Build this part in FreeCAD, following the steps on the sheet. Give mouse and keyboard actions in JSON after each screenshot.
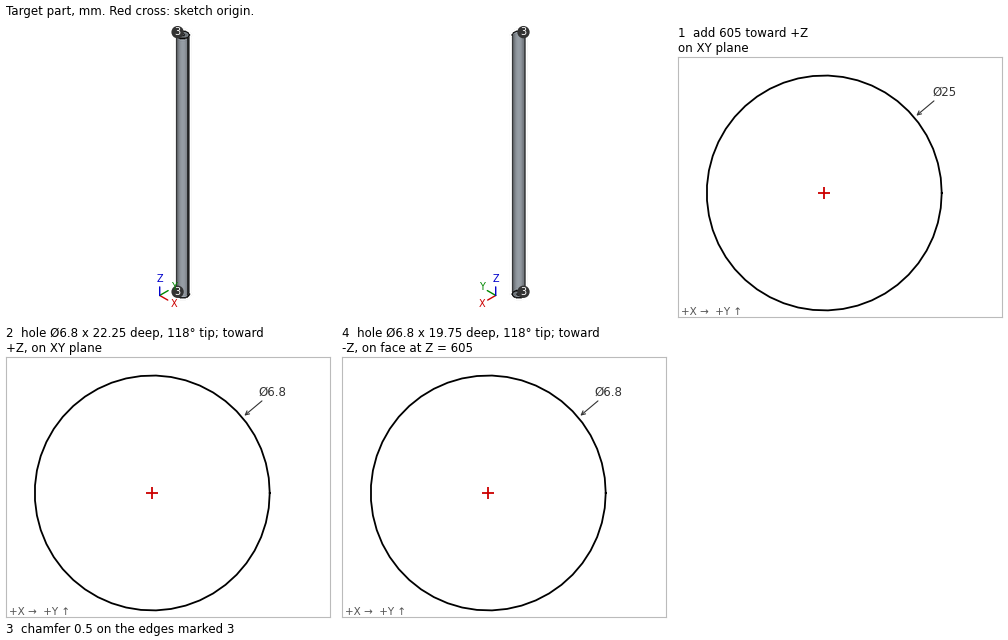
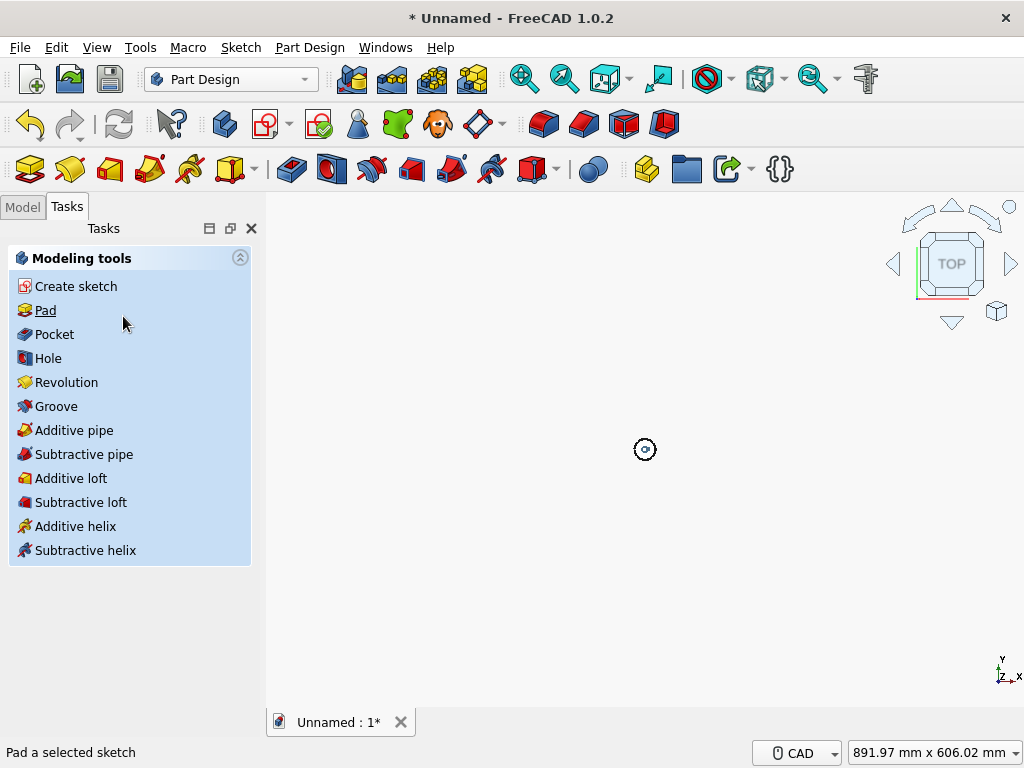
{"action": "left_click", "coordinate": [332, 170]}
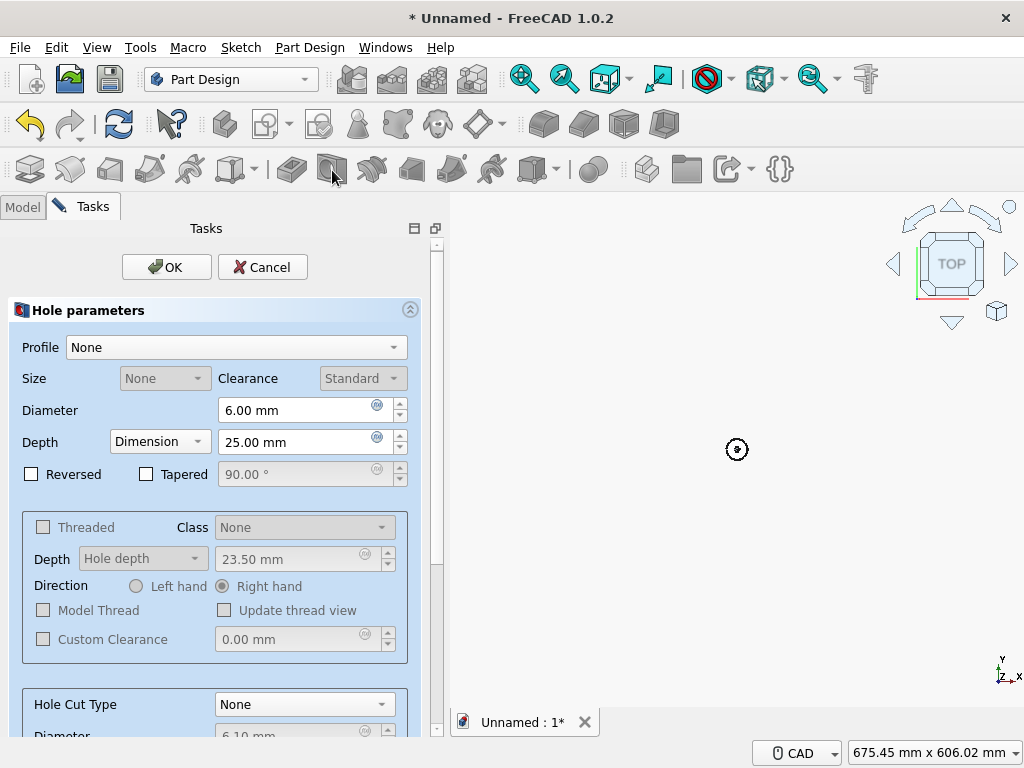
{"action": "triple_click", "coordinate": [305, 410]}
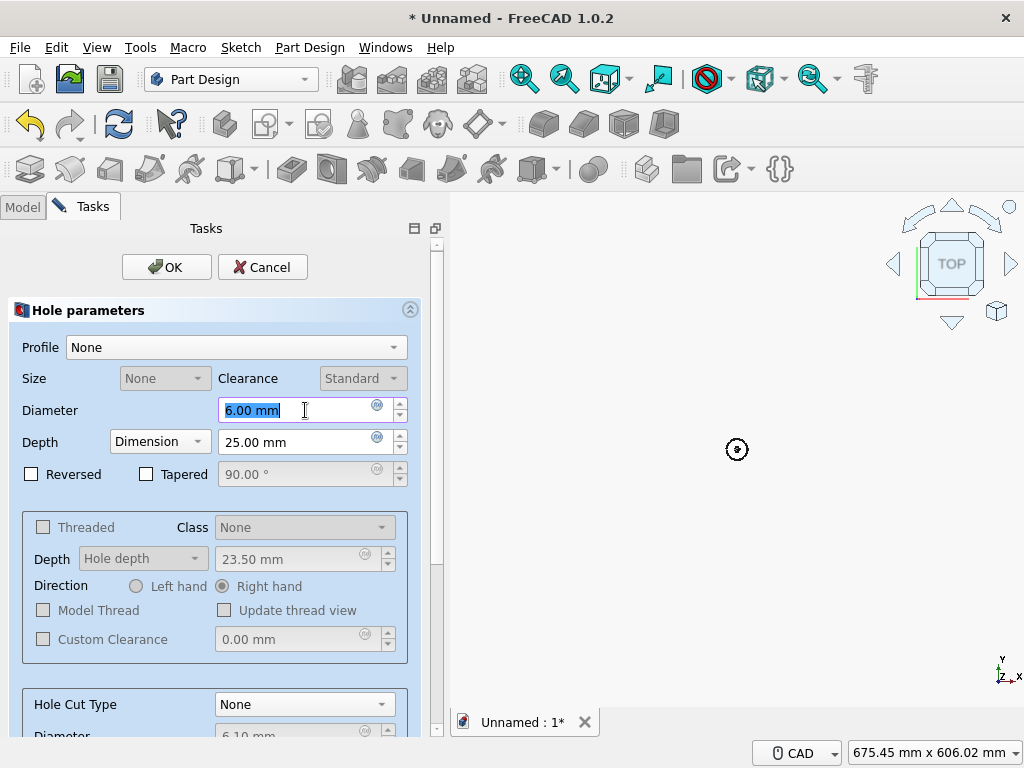
{"action": "type", "text": "6.8"}
{"action": "key", "text": "Tab"}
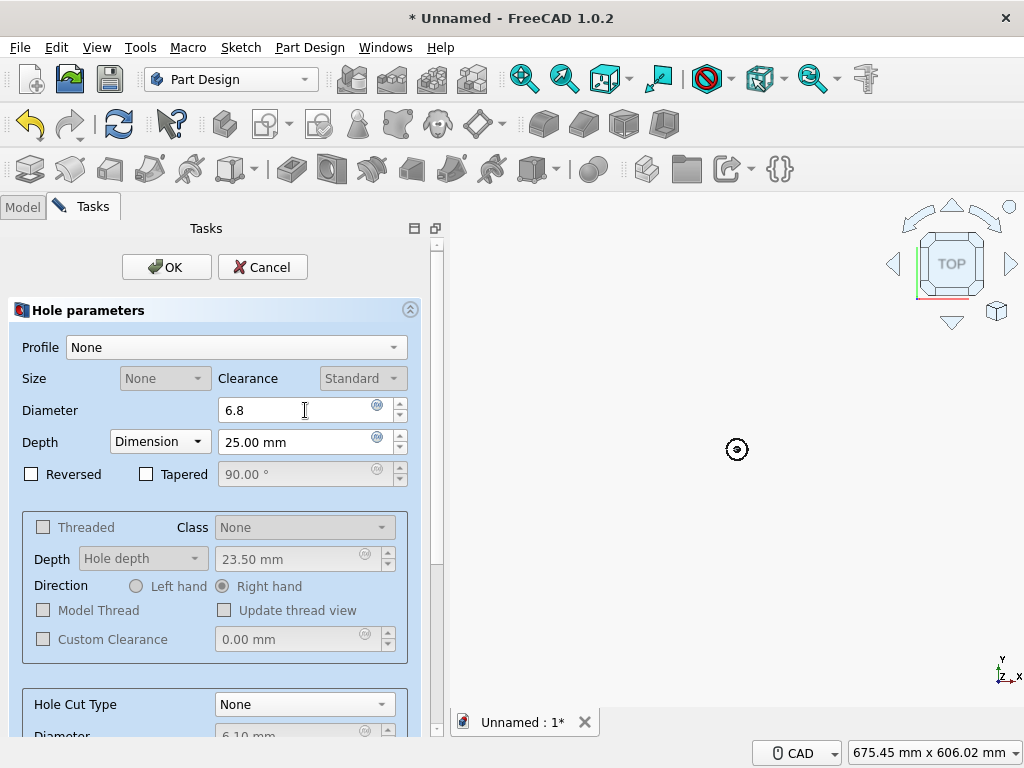
{"action": "triple_click", "coordinate": [305, 442]}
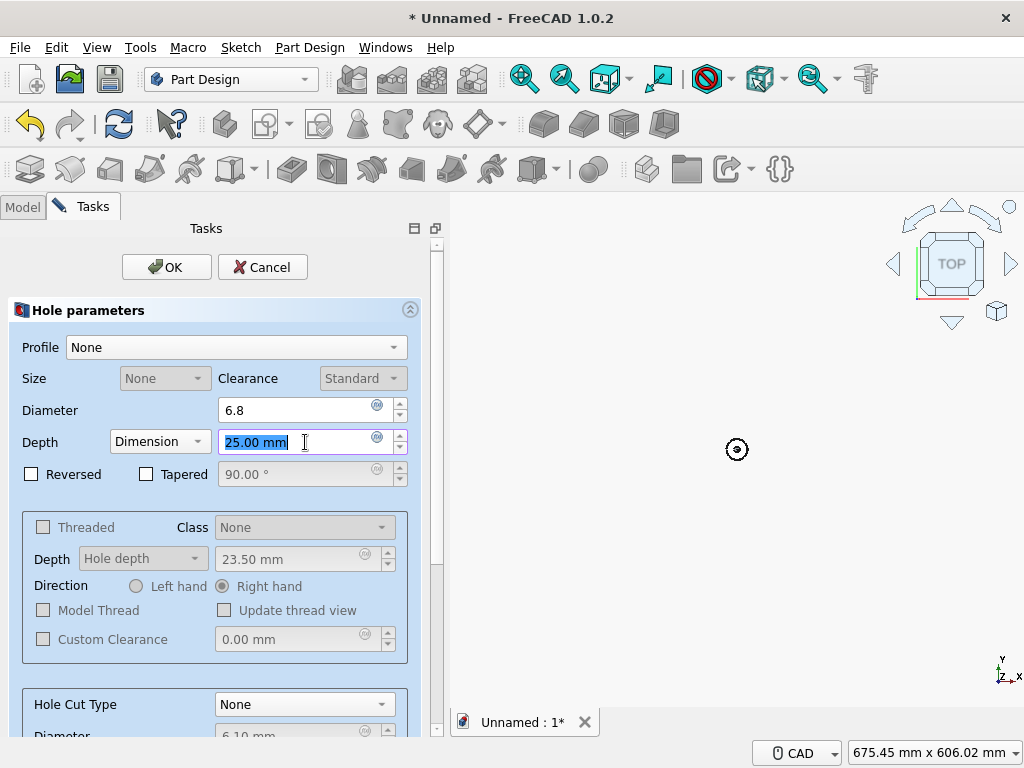
{"action": "type", "text": "19.75"}
{"action": "key", "text": "Tab"}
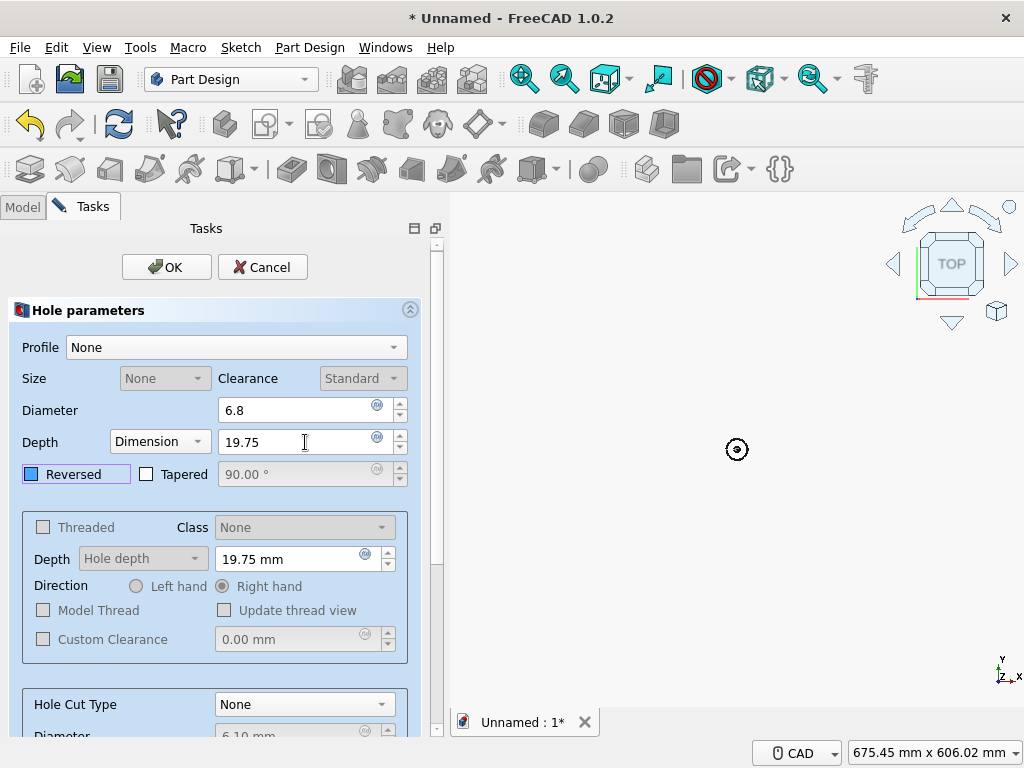
{"action": "left_click", "coordinate": [167, 267]}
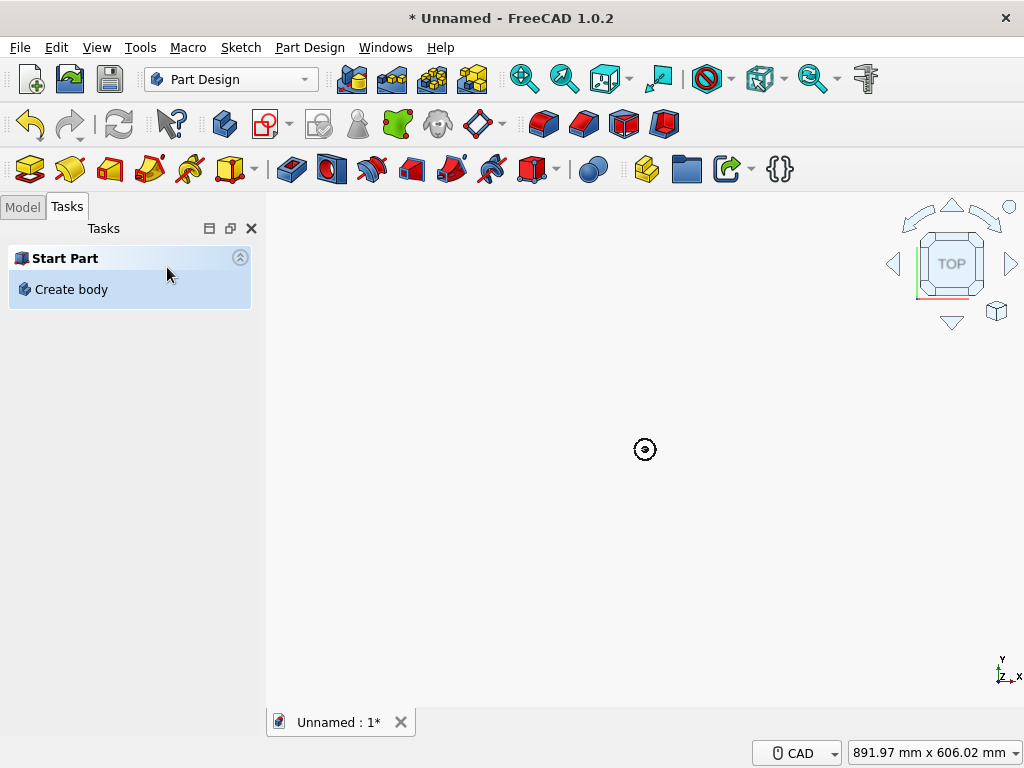
{"action": "key", "text": "0"}